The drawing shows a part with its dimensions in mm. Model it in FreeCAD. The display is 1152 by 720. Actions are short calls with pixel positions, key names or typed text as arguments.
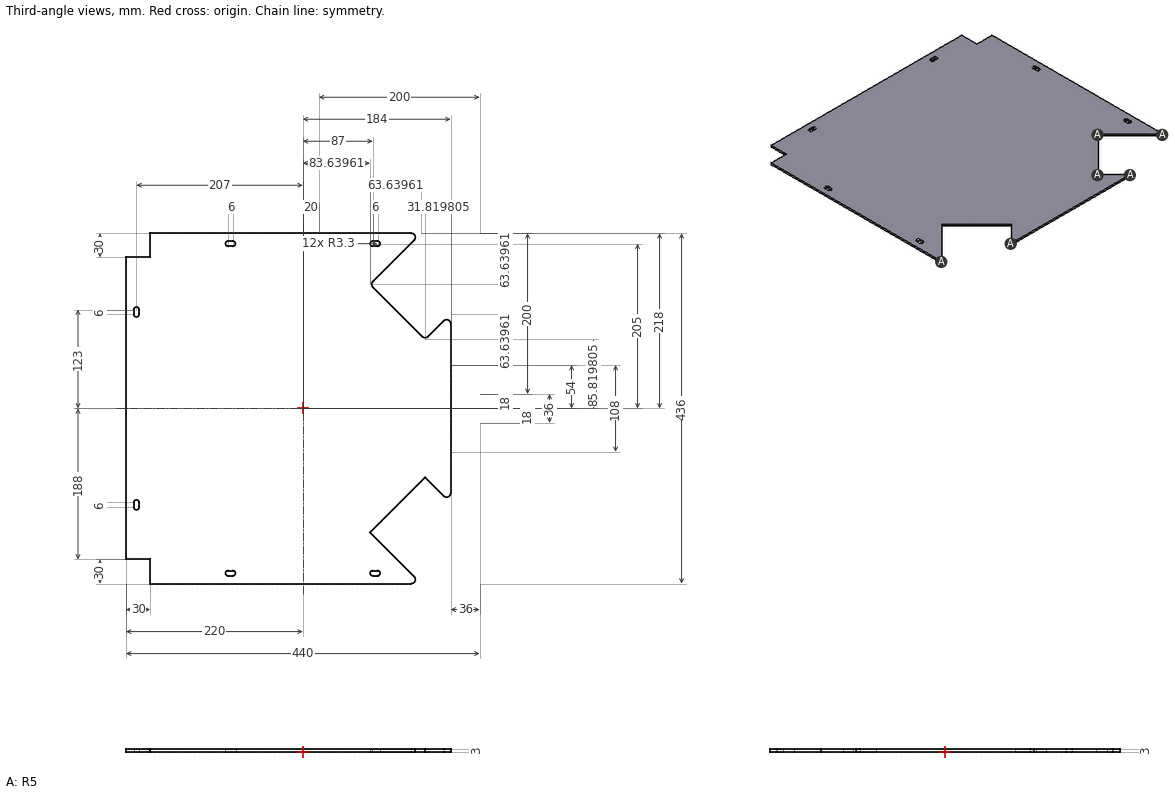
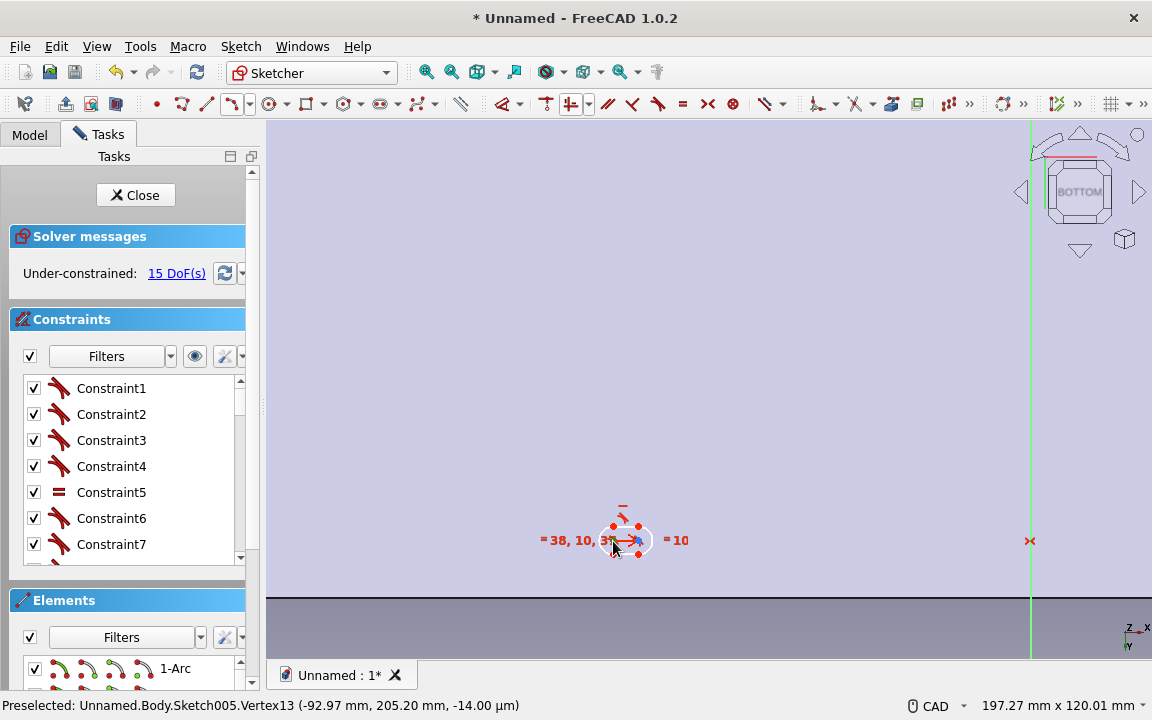
scroll(614, 542, down, 9)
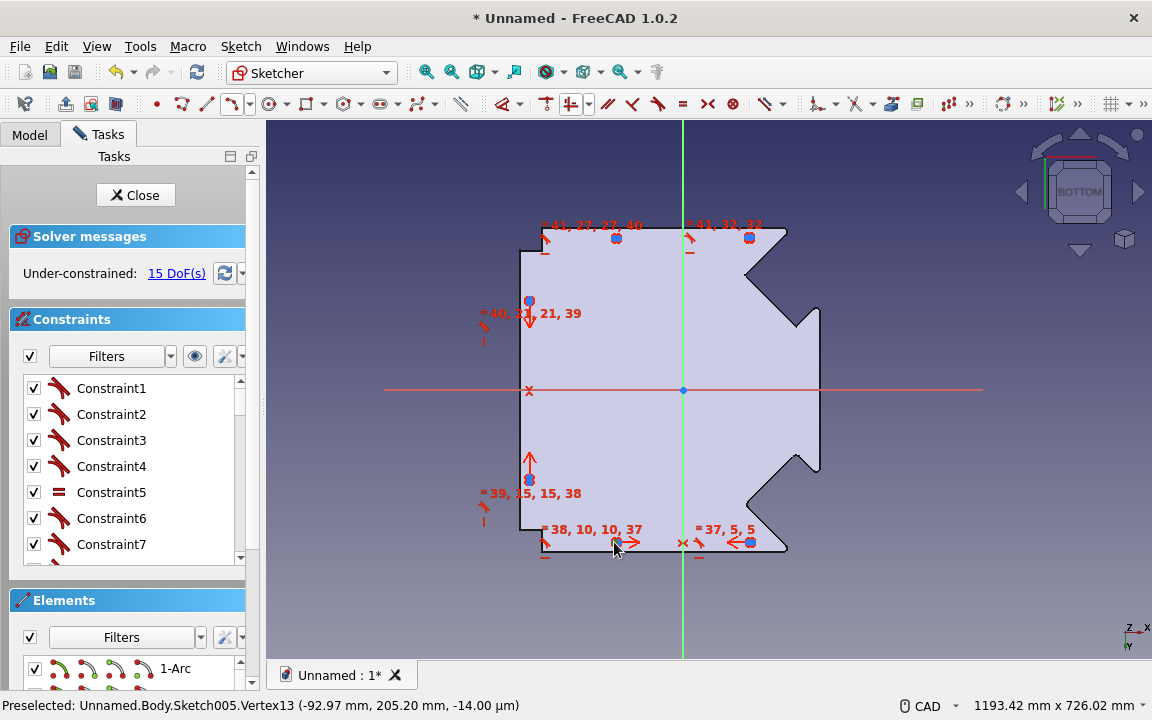
scroll(614, 239, up, 9)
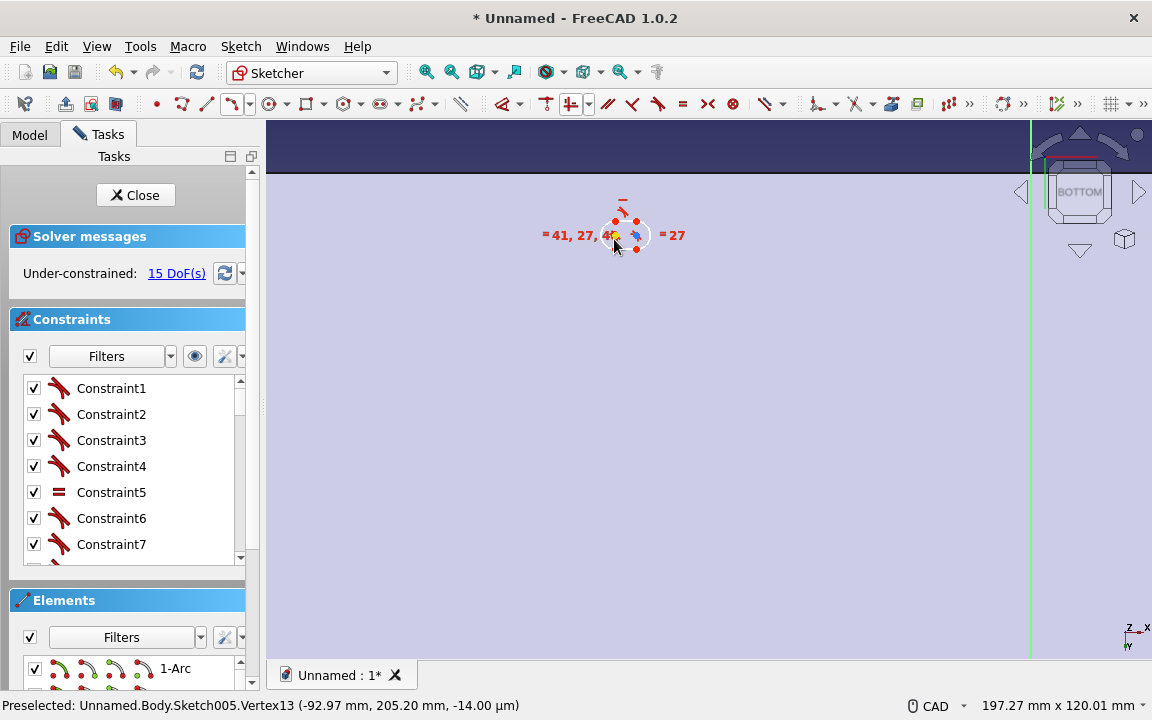
click(615, 235)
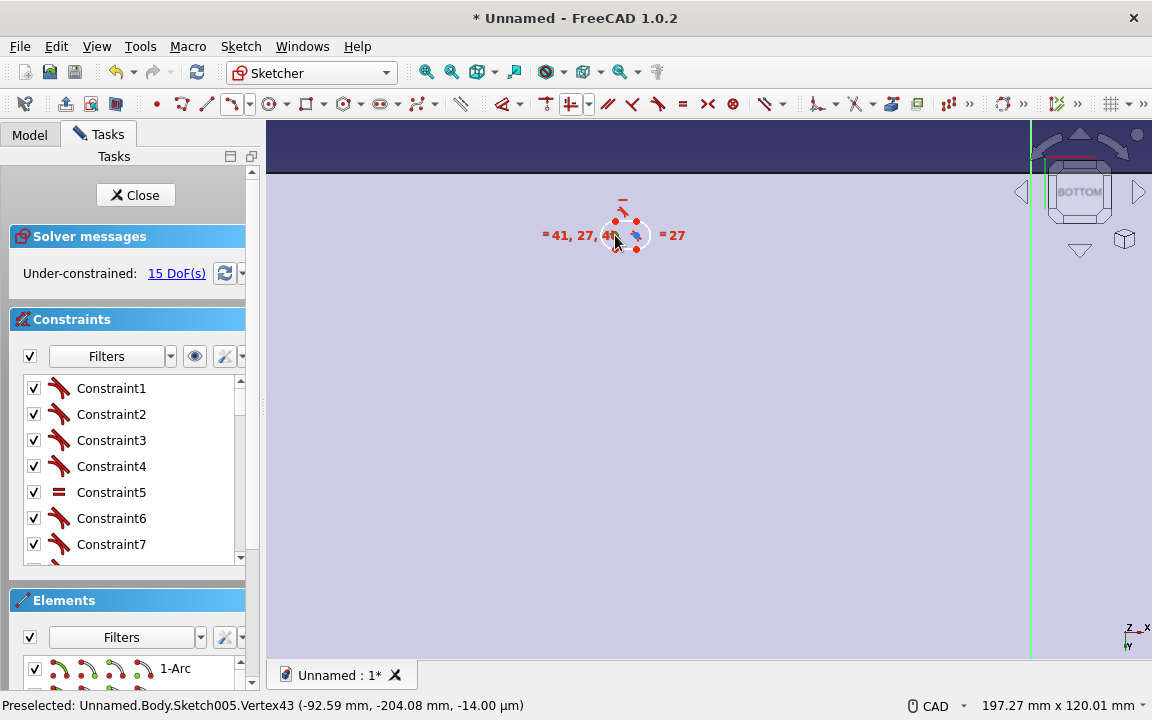
scroll(614, 239, down, 9)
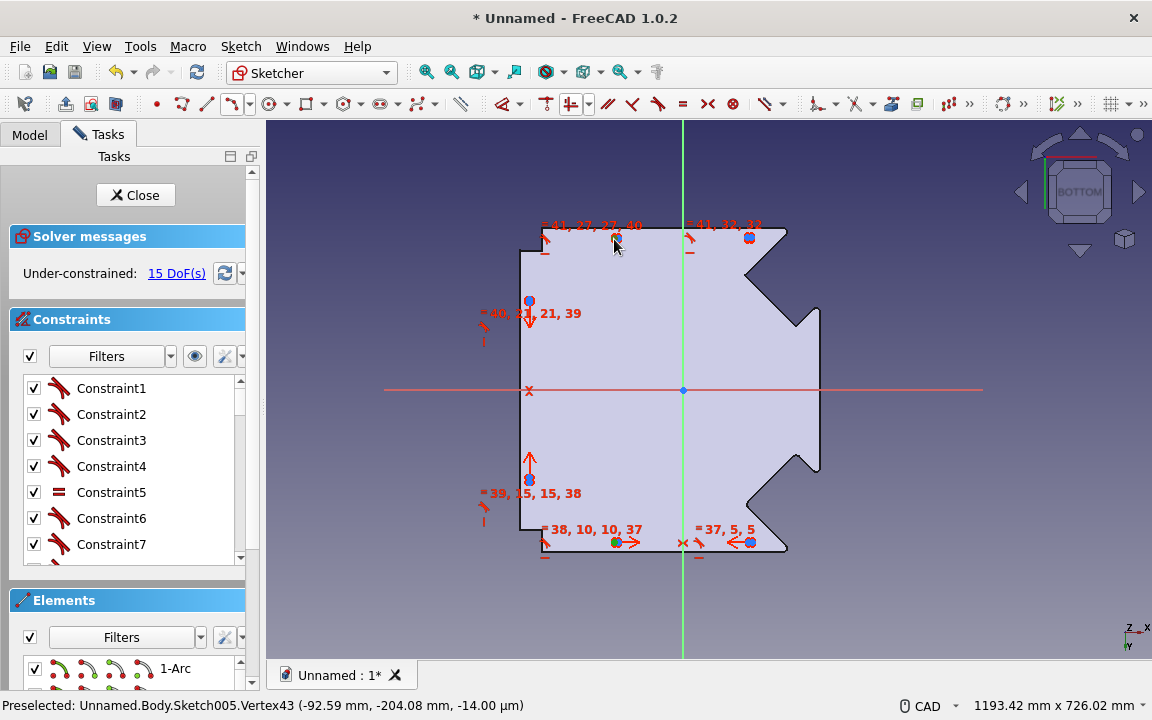
click(393, 390)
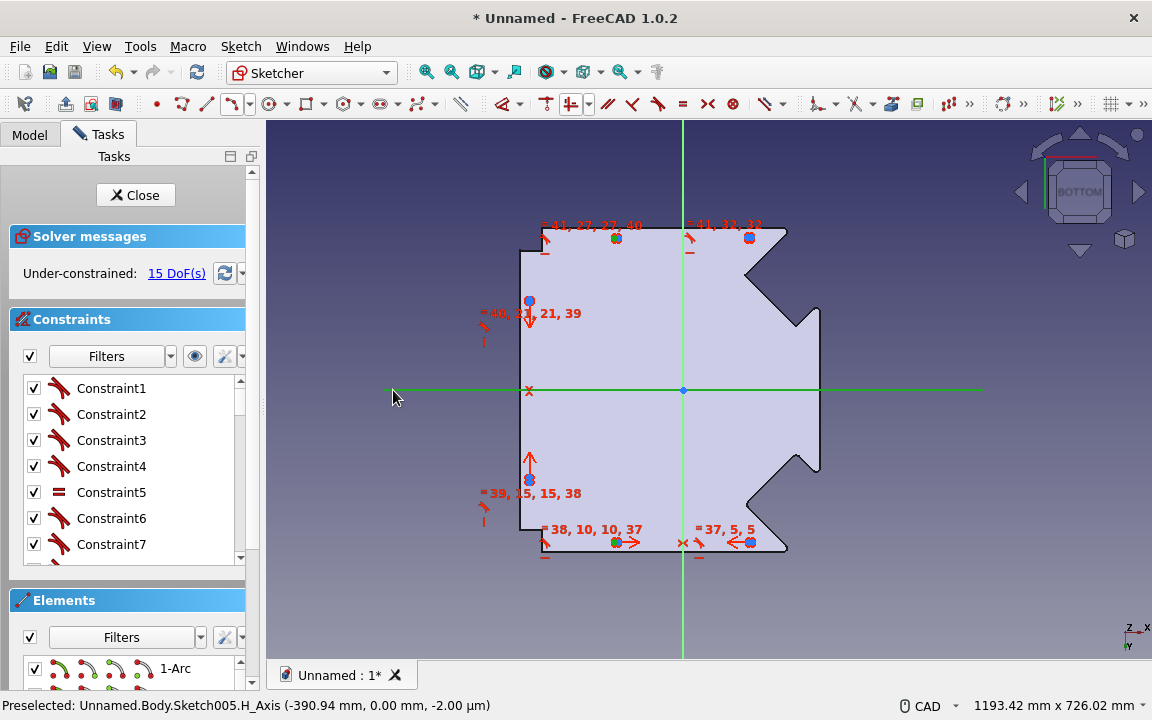
click(708, 104)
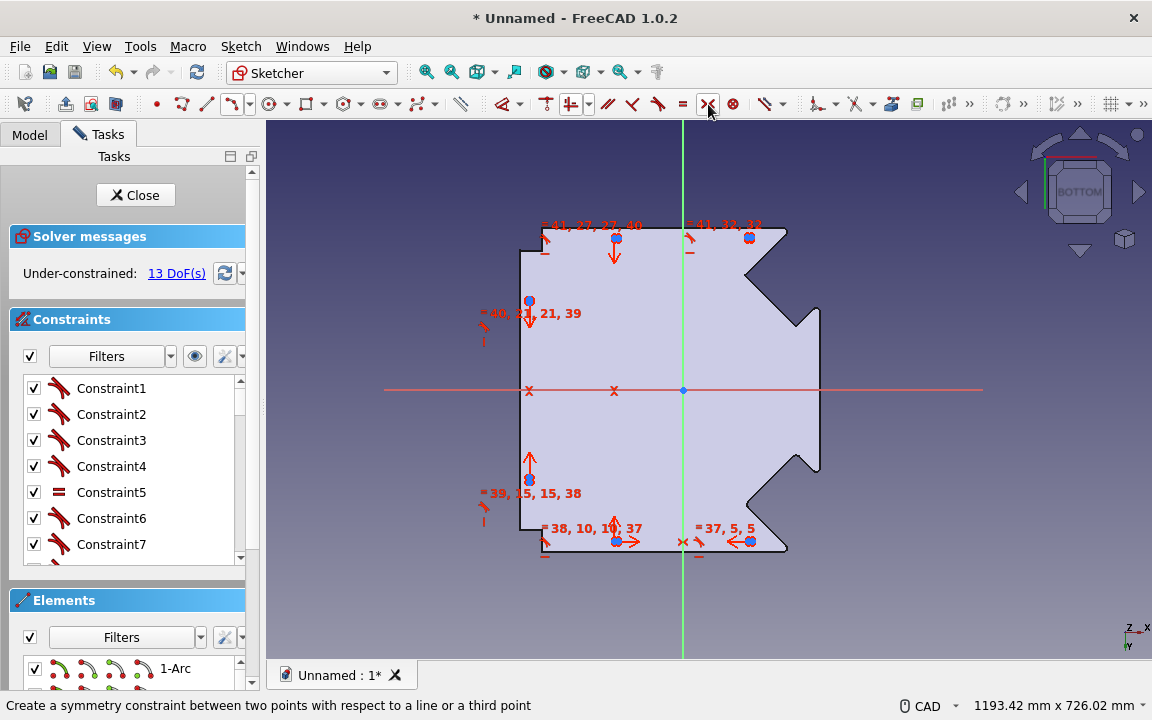
scroll(748, 542, up, 9)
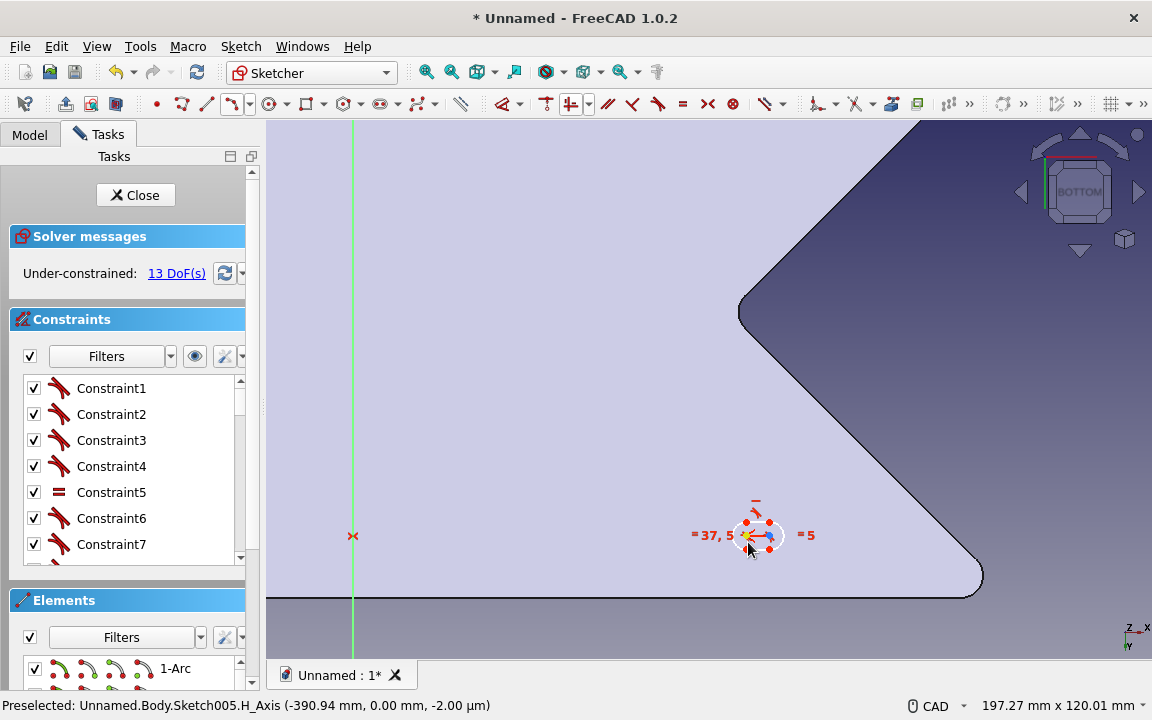
click(747, 536)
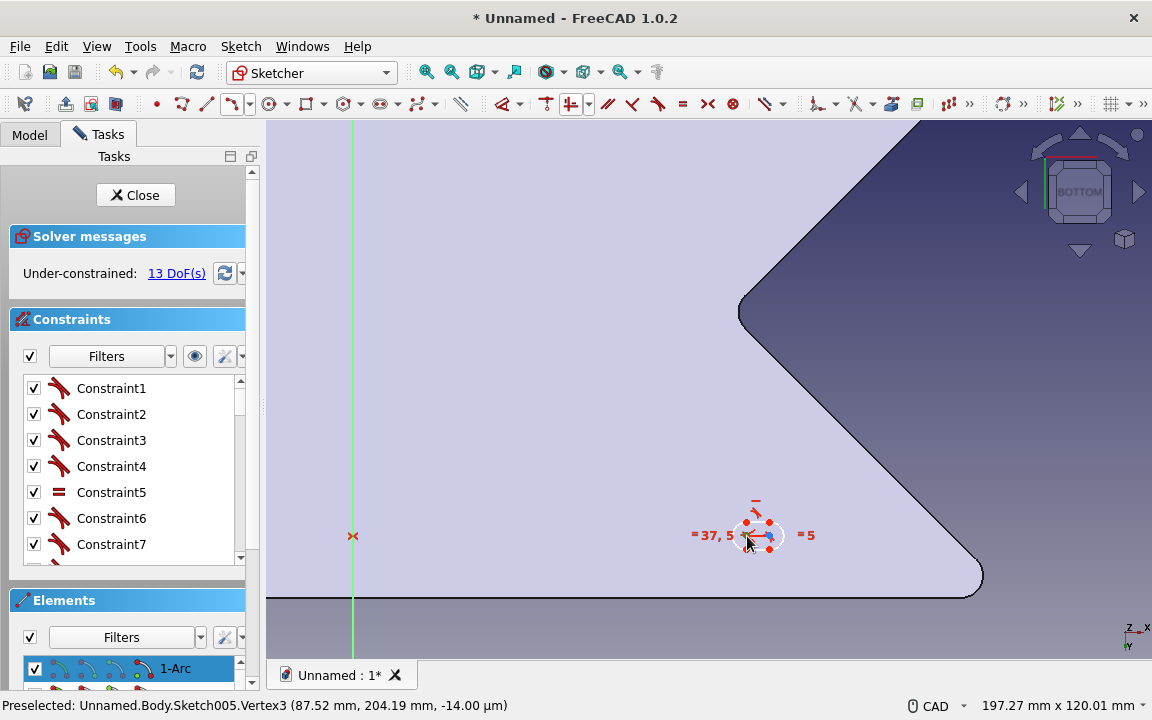
scroll(748, 542, down, 9)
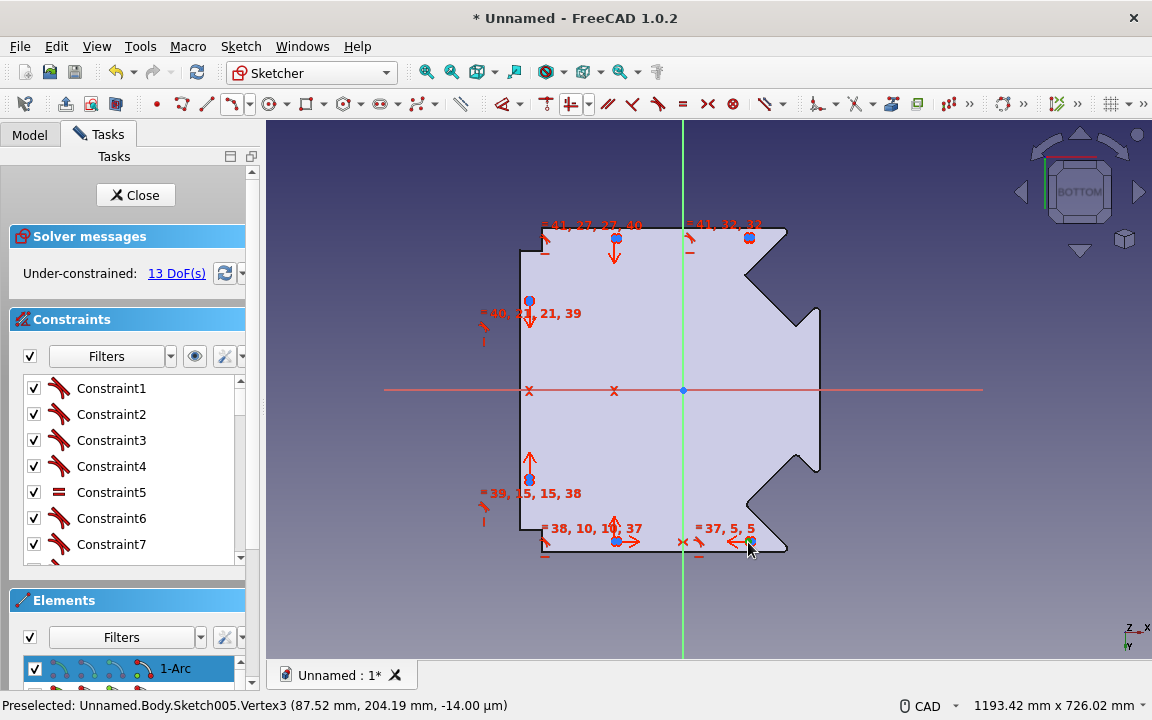
scroll(748, 238, up, 9)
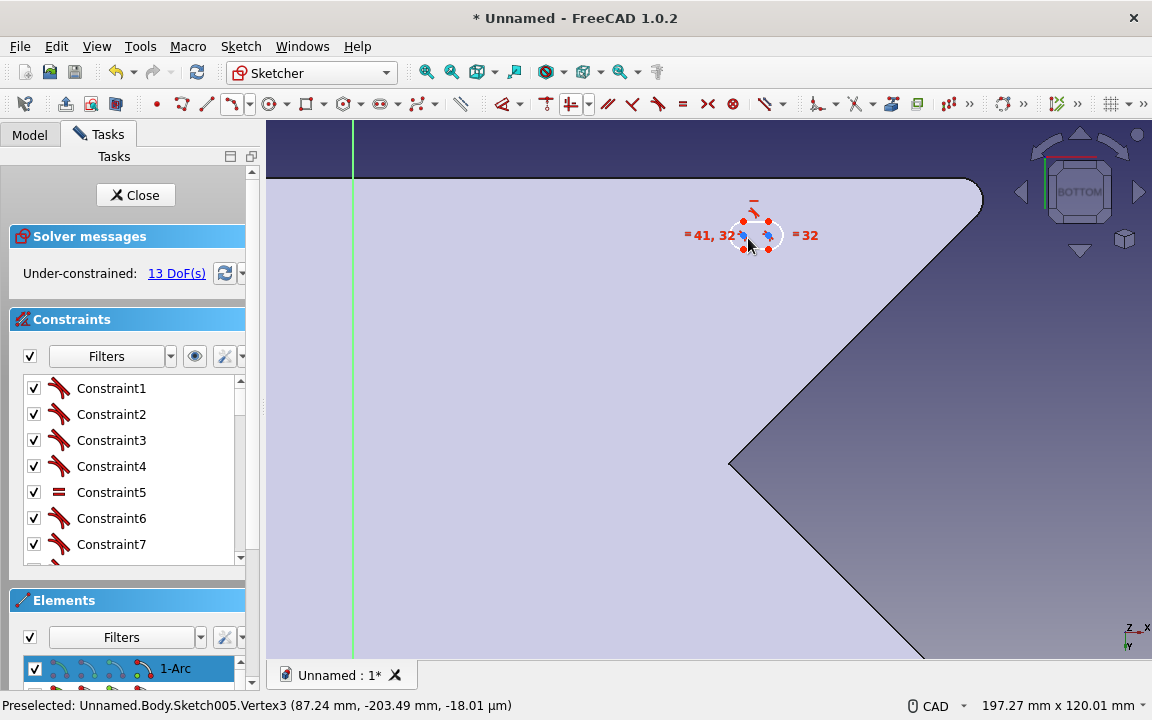
click(744, 235)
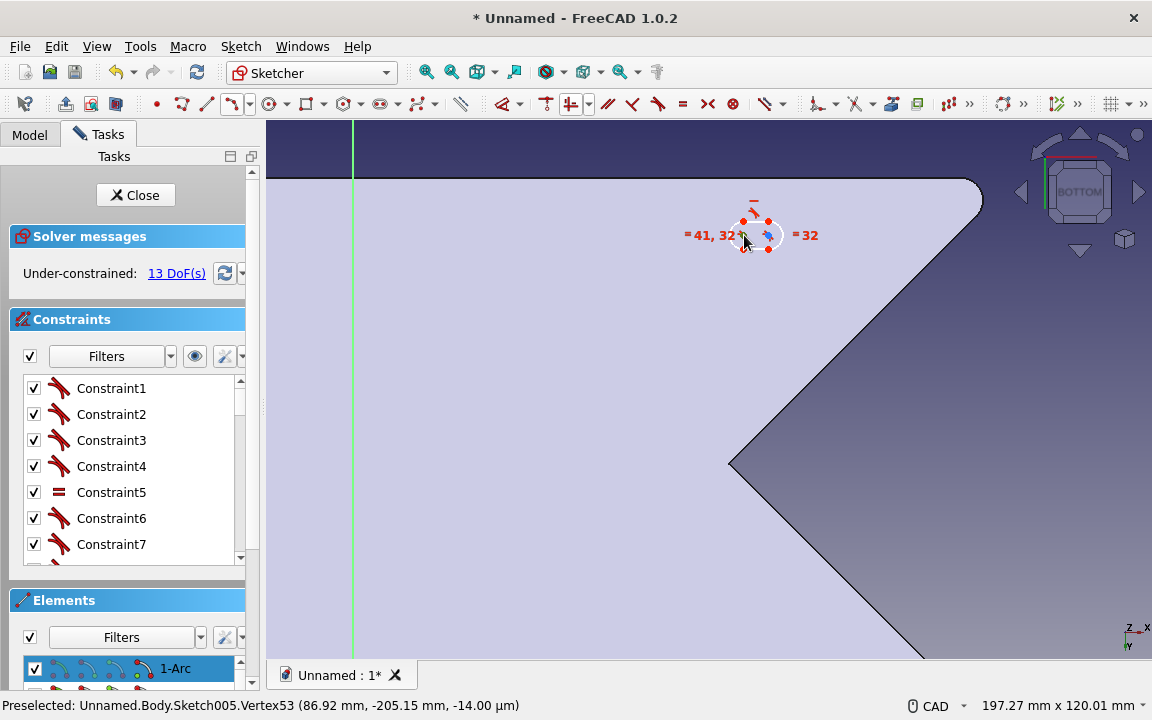
scroll(748, 238, down, 9)